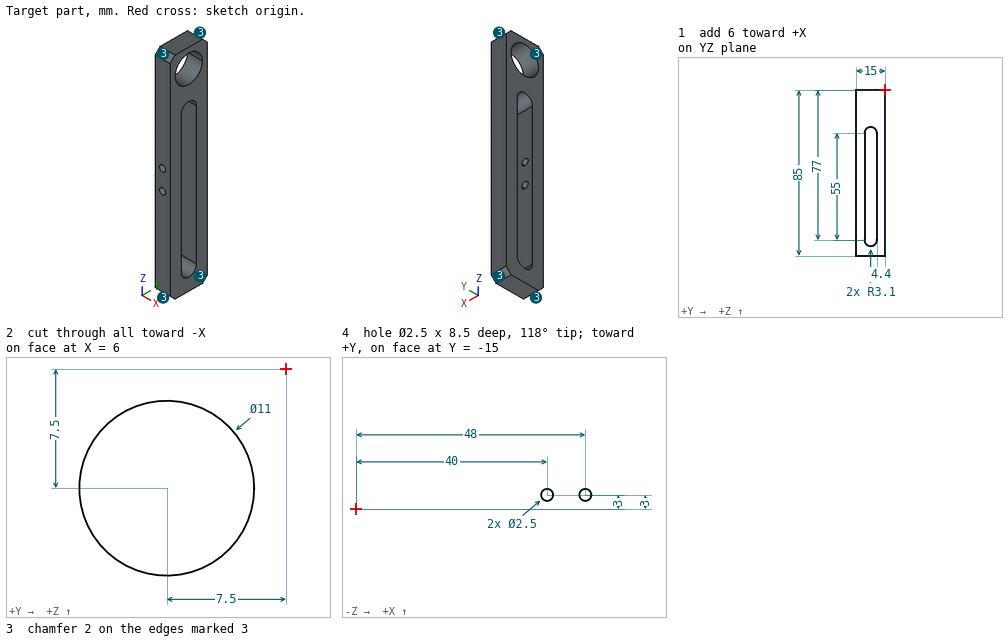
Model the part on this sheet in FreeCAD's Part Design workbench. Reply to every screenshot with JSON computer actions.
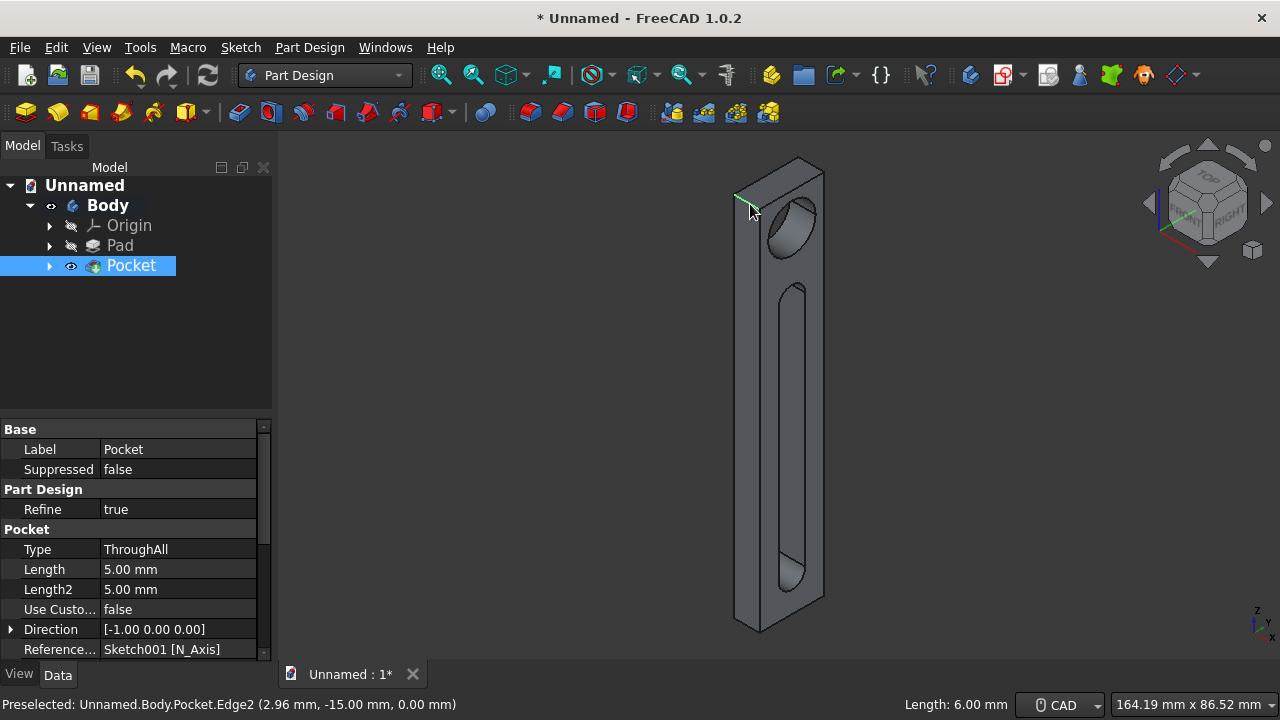
{"action": "key", "text": "2"}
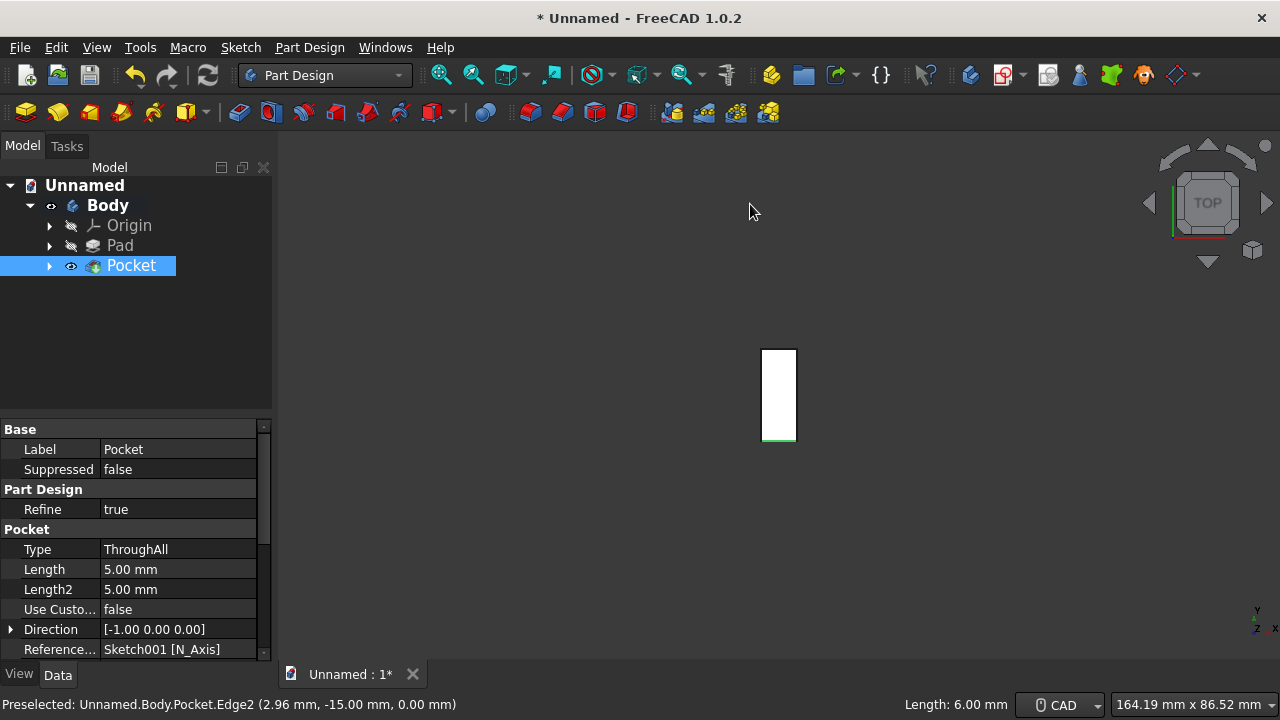
{"action": "key", "text": "v f"}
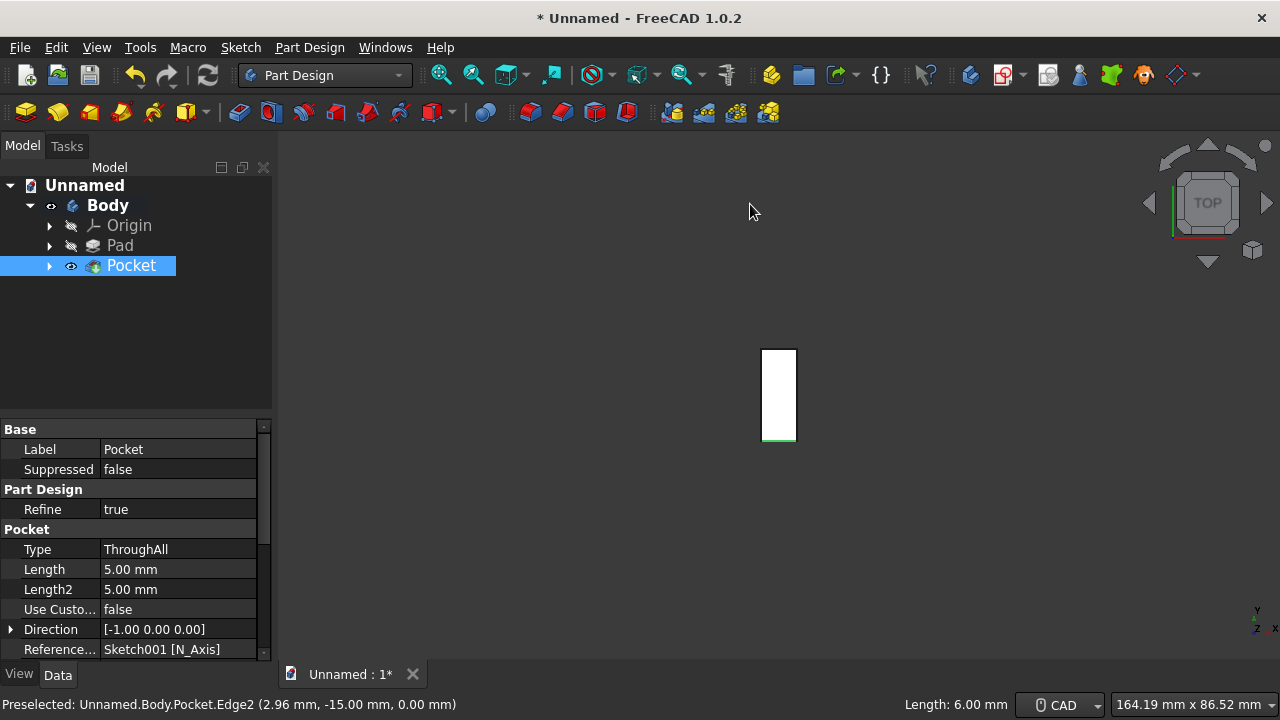
{"action": "key", "text": "1"}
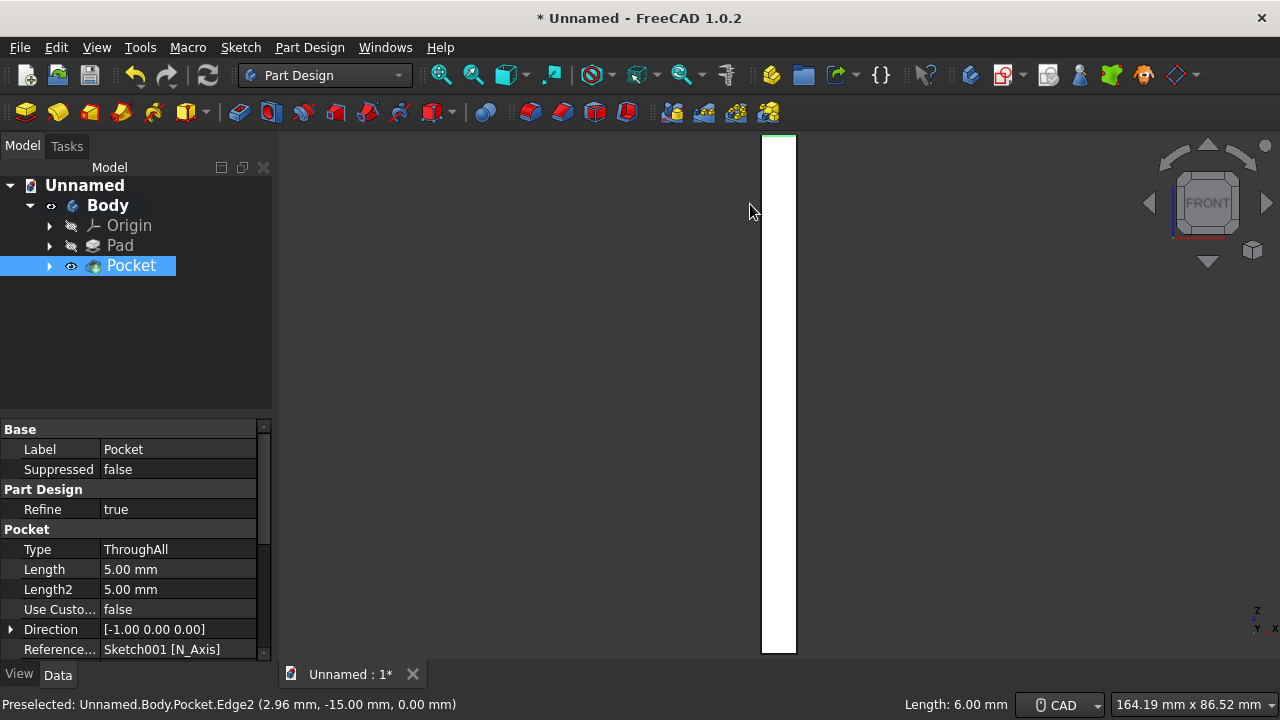
{"action": "key", "text": "3"}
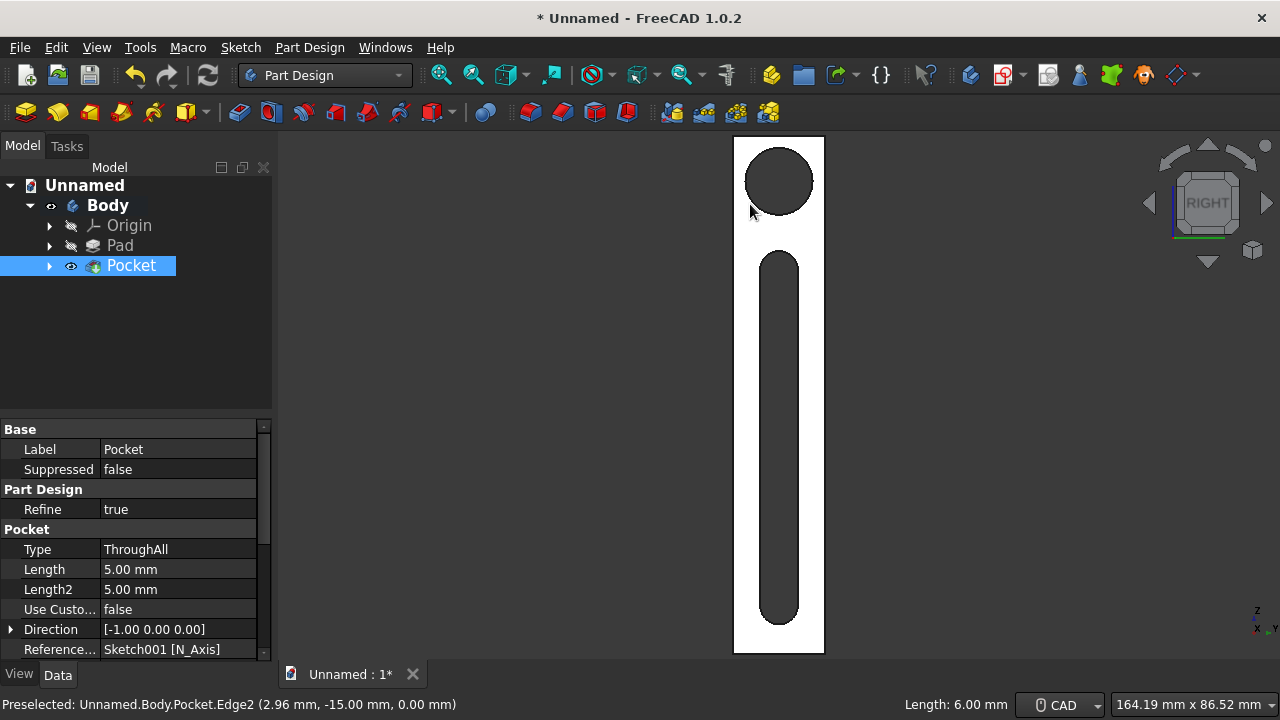
{"action": "key", "text": "5"}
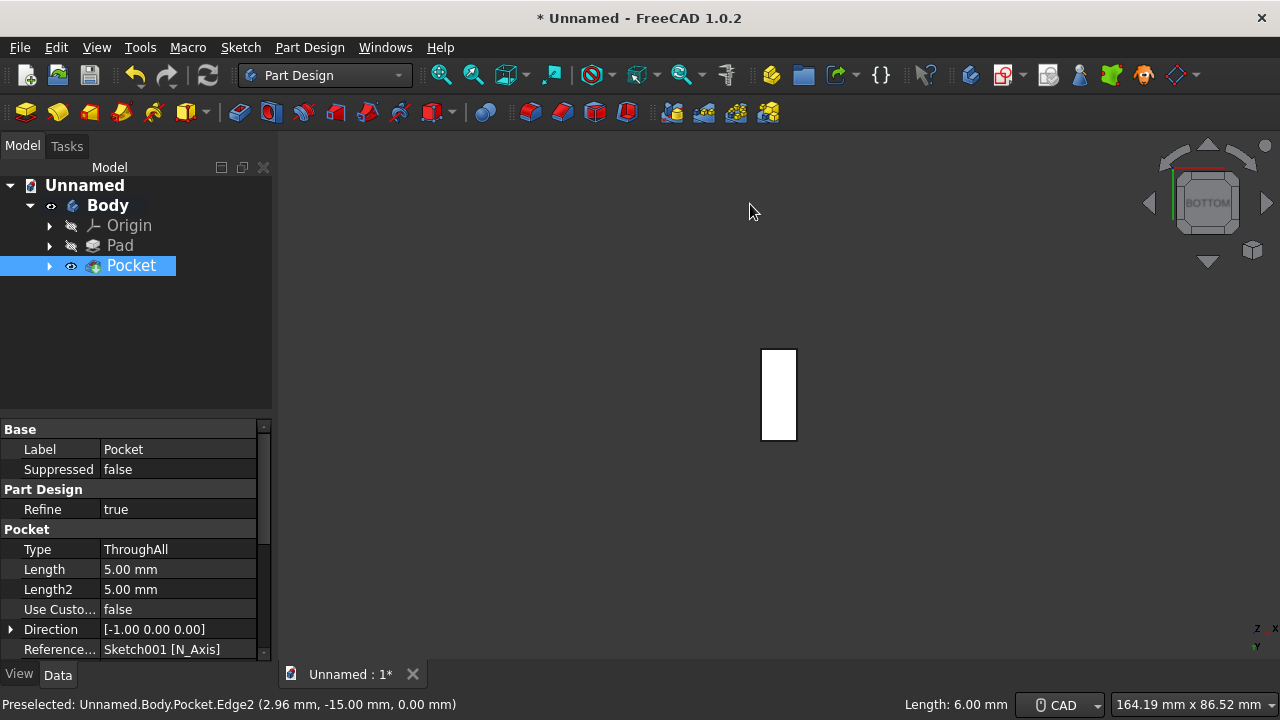
{"action": "key", "text": "v f"}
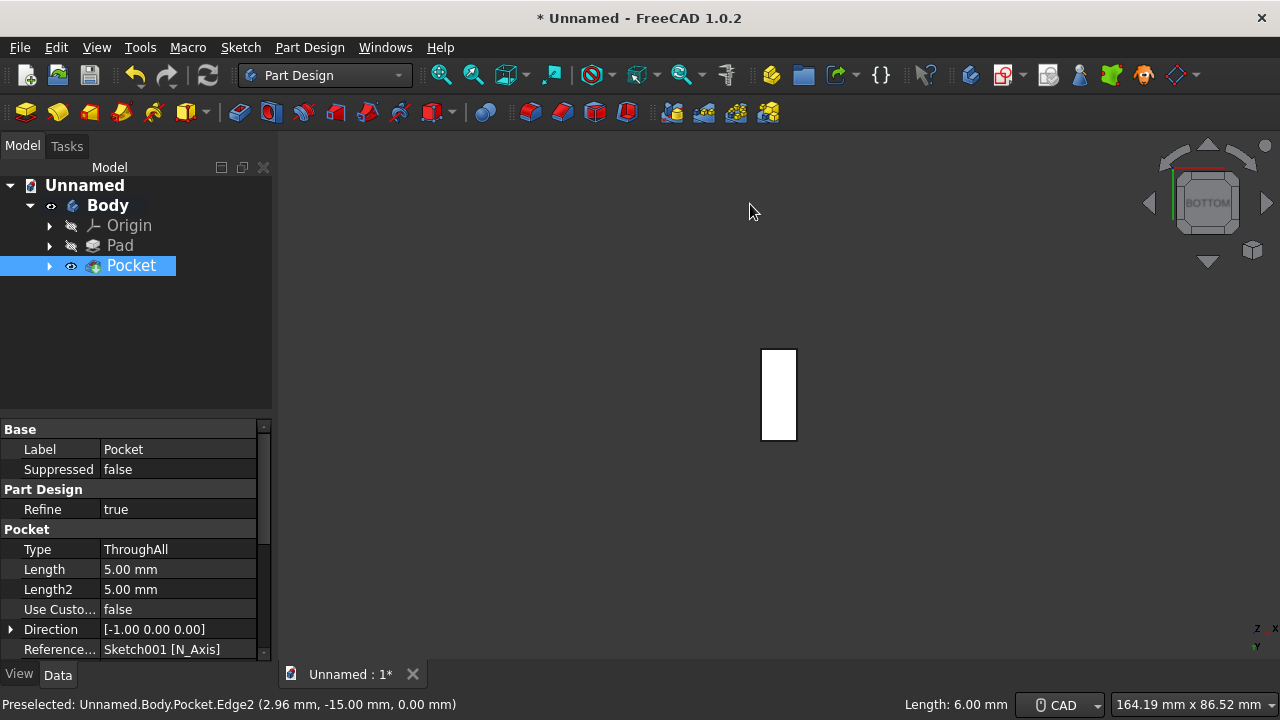
{"action": "left_click", "coordinate": [779, 440], "text": "ctrl"}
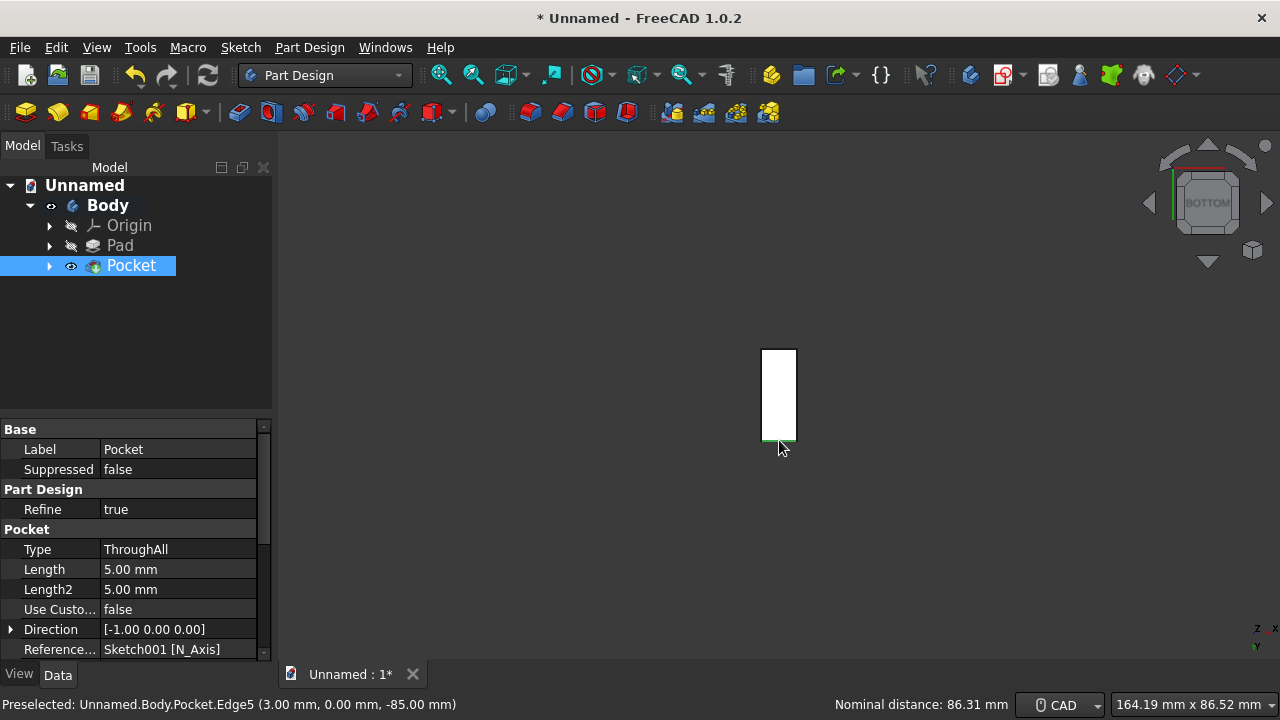
{"action": "left_click", "coordinate": [779, 348], "text": "ctrl"}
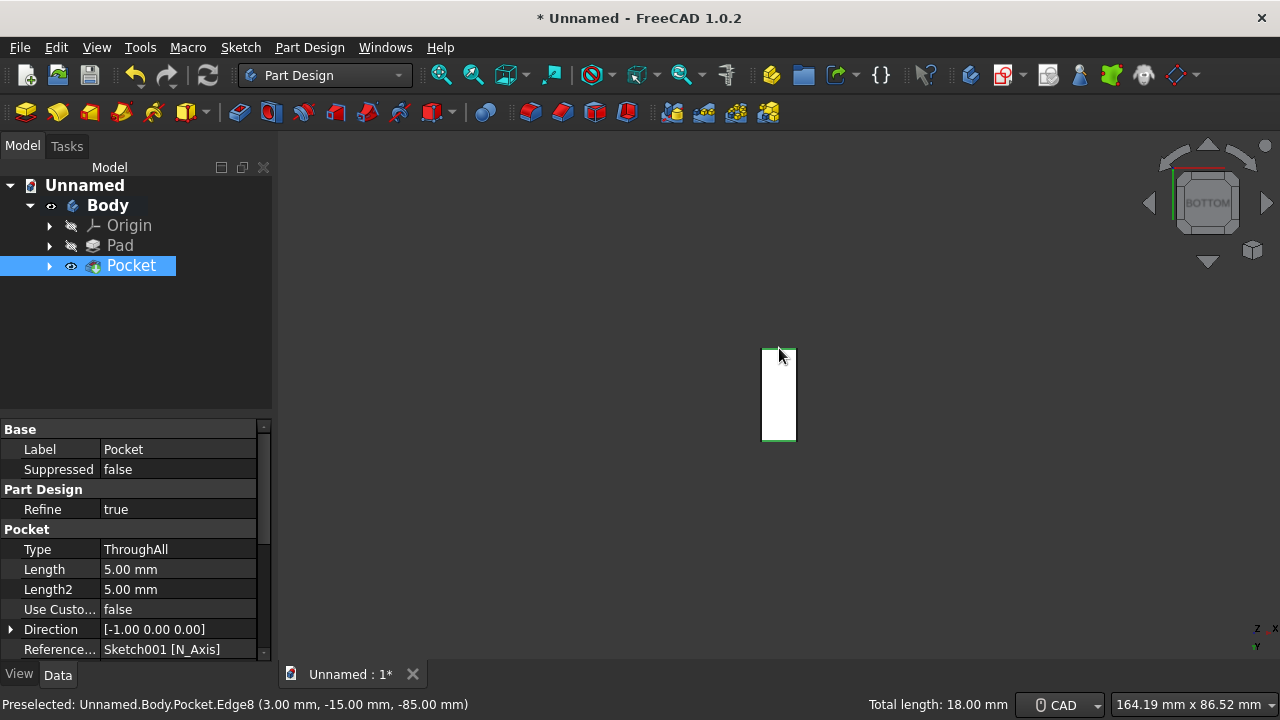
{"action": "key", "text": "4"}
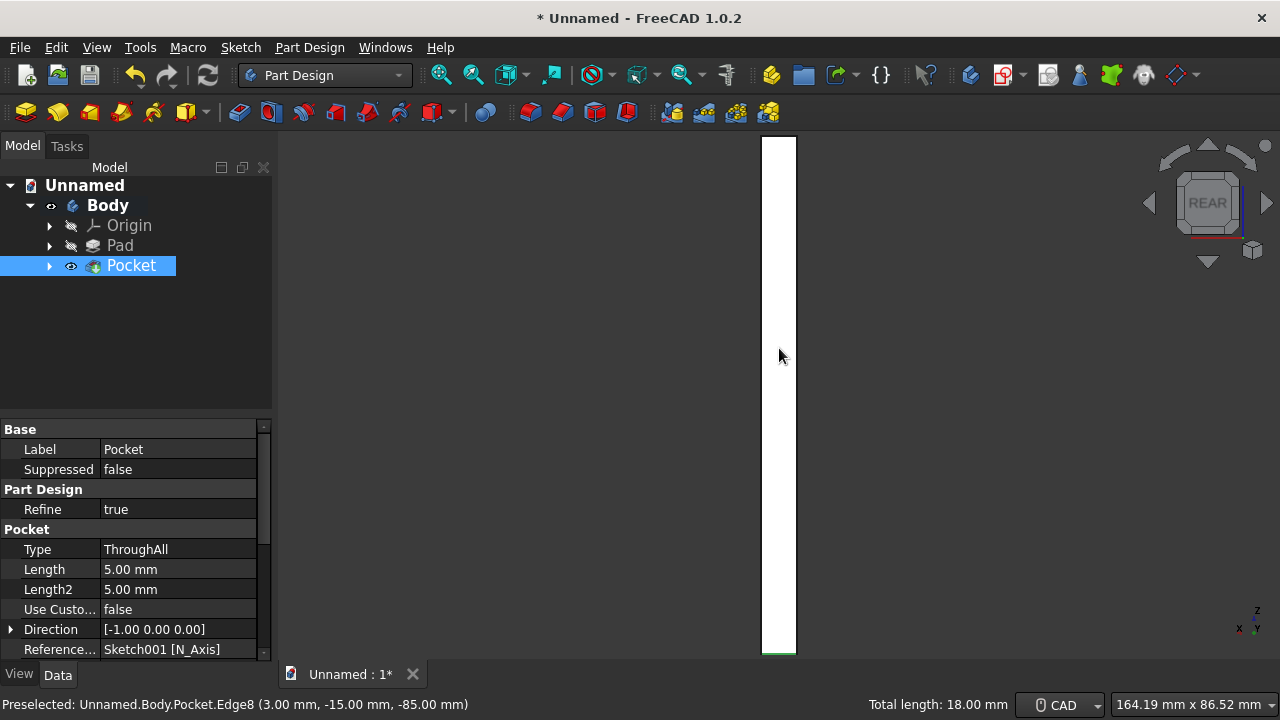
{"action": "key", "text": "6"}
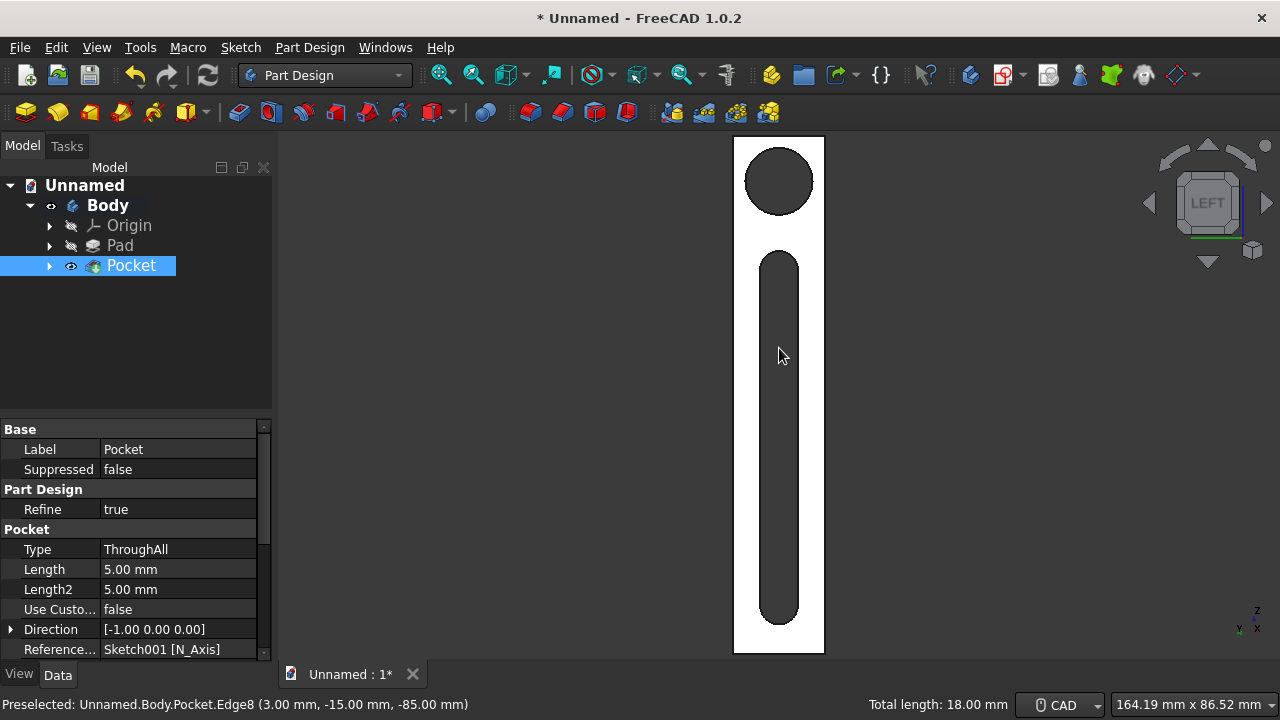
{"action": "key", "text": "v 3"}